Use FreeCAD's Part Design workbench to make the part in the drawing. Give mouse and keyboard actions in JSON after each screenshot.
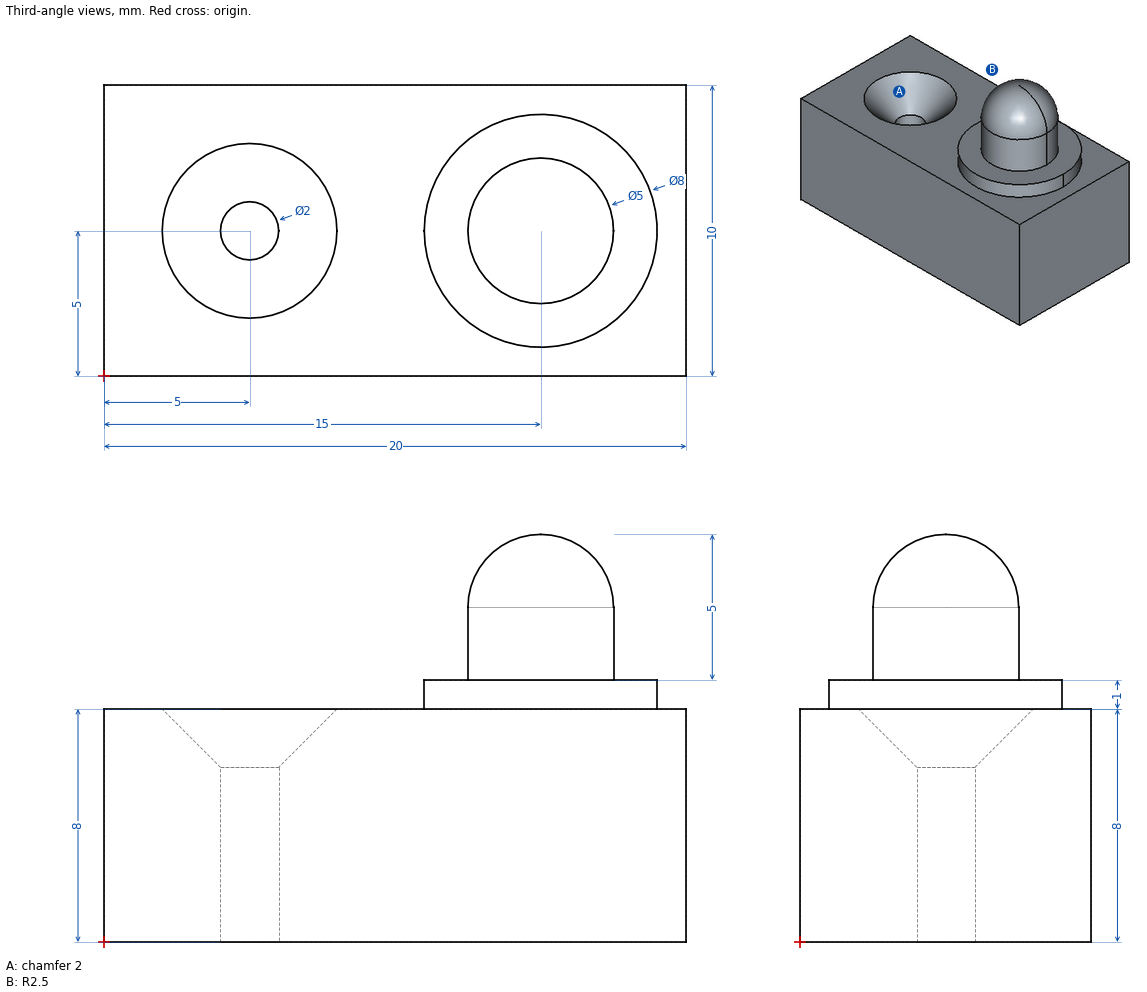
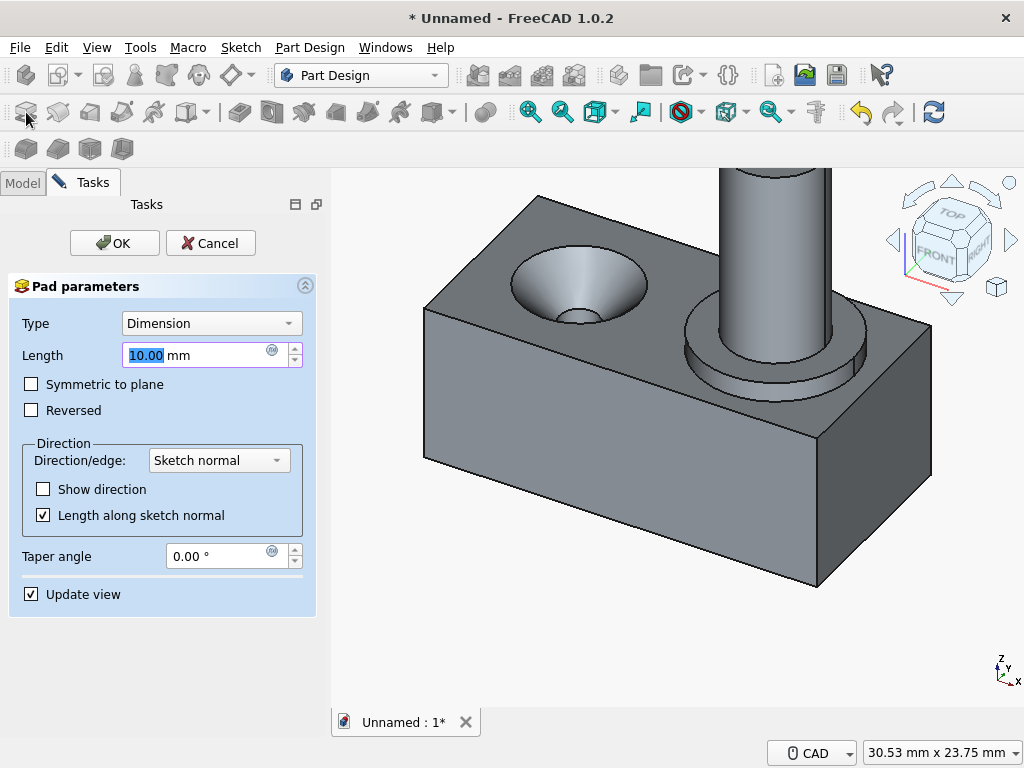
{"action": "type", "text": "5"}
{"action": "key", "text": "Tab"}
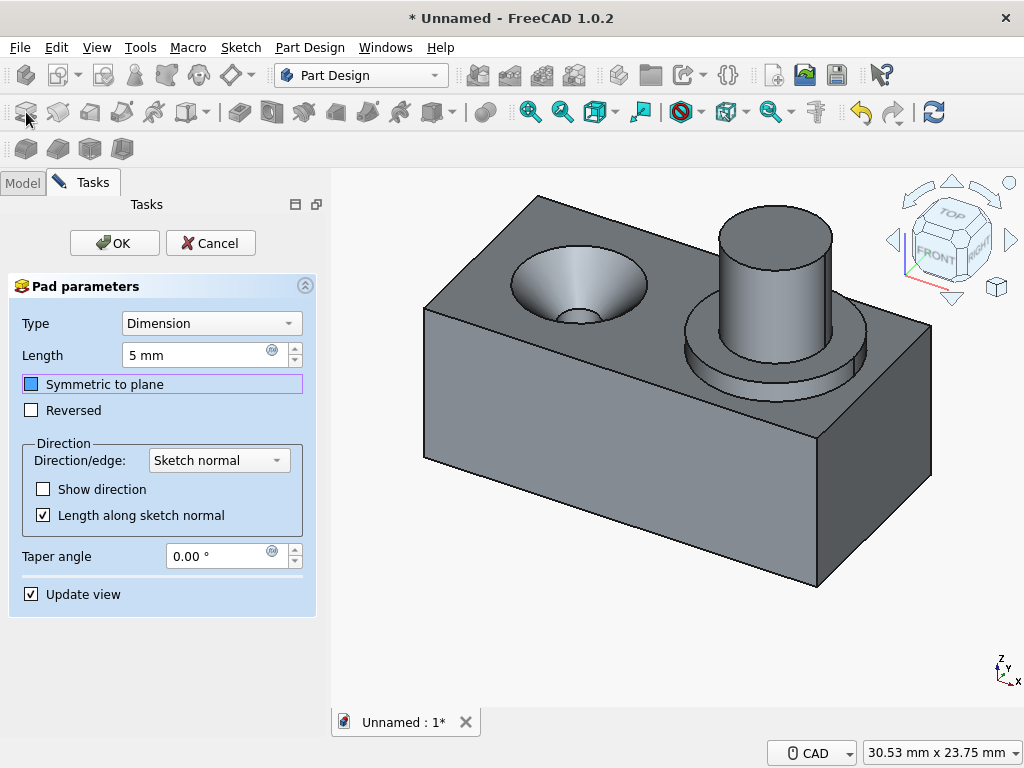
{"action": "left_click", "coordinate": [115, 243]}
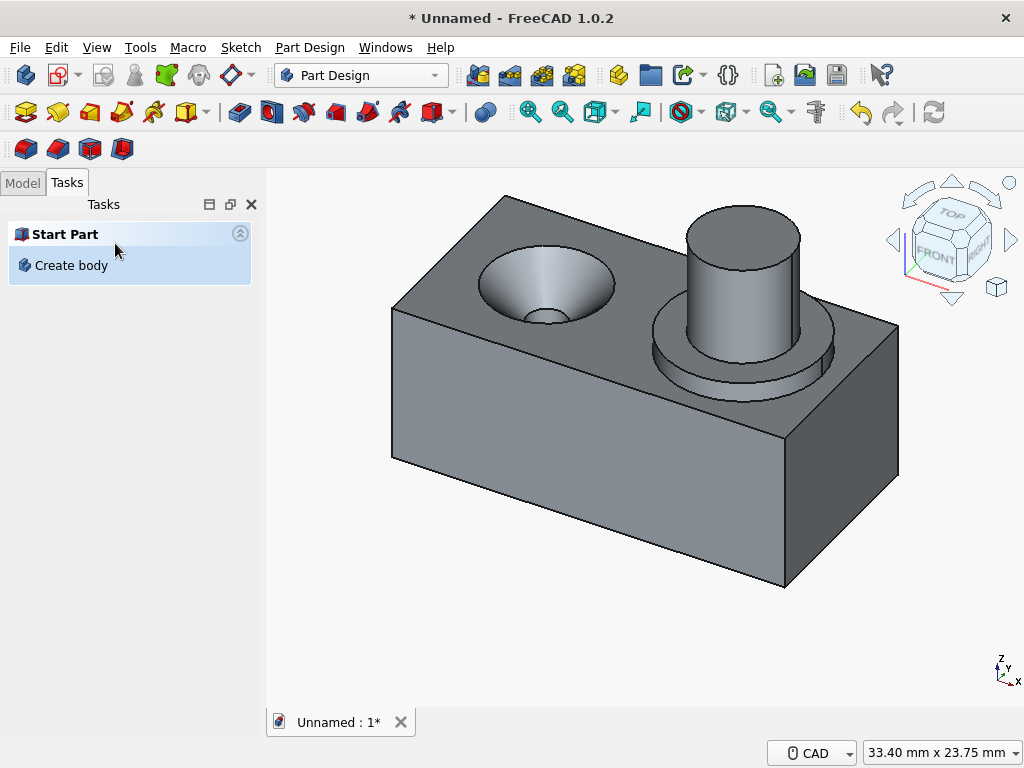
{"action": "left_click", "coordinate": [532, 112]}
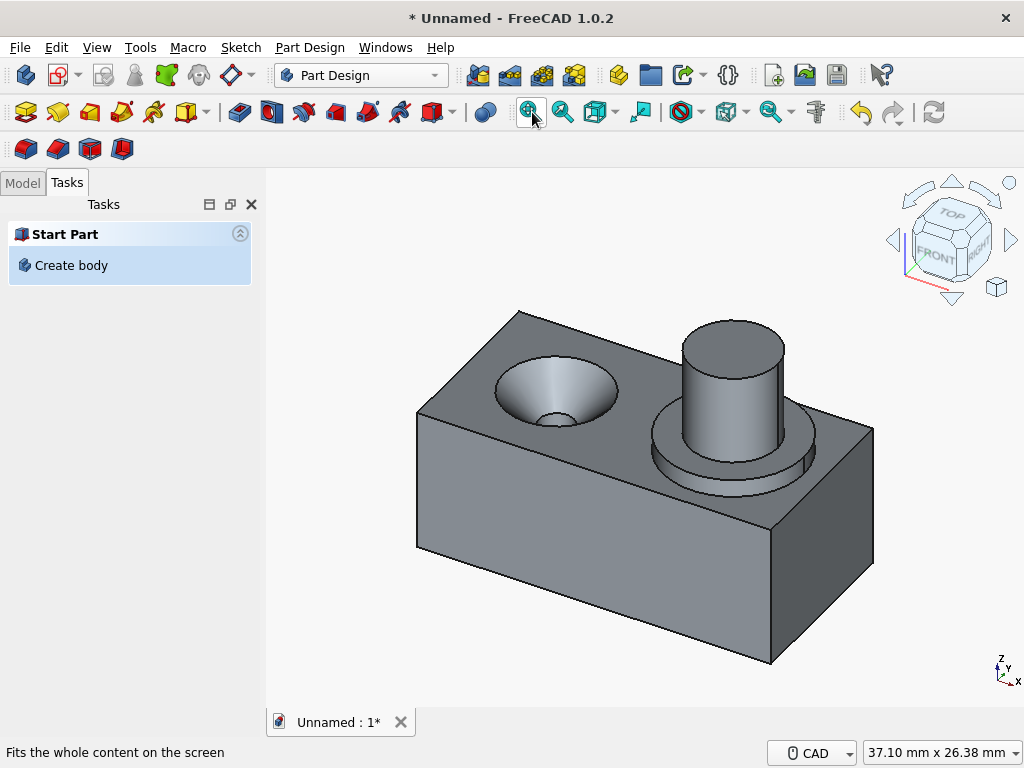
{"action": "left_click", "coordinate": [683, 352]}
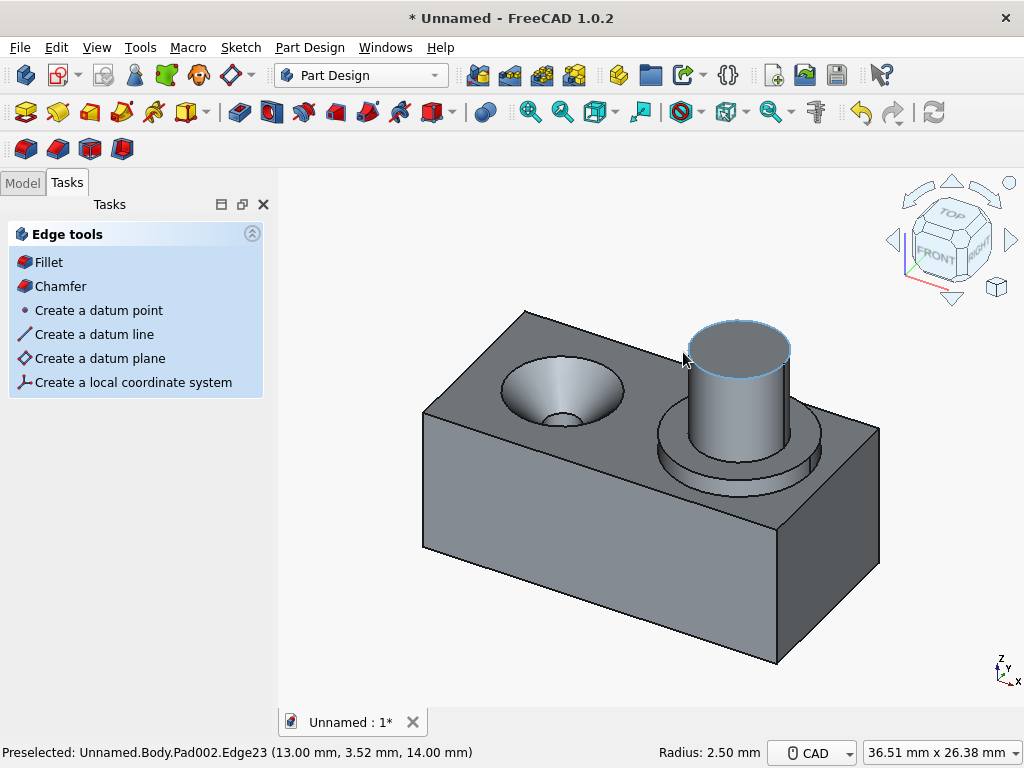
{"action": "left_click", "coordinate": [26, 150]}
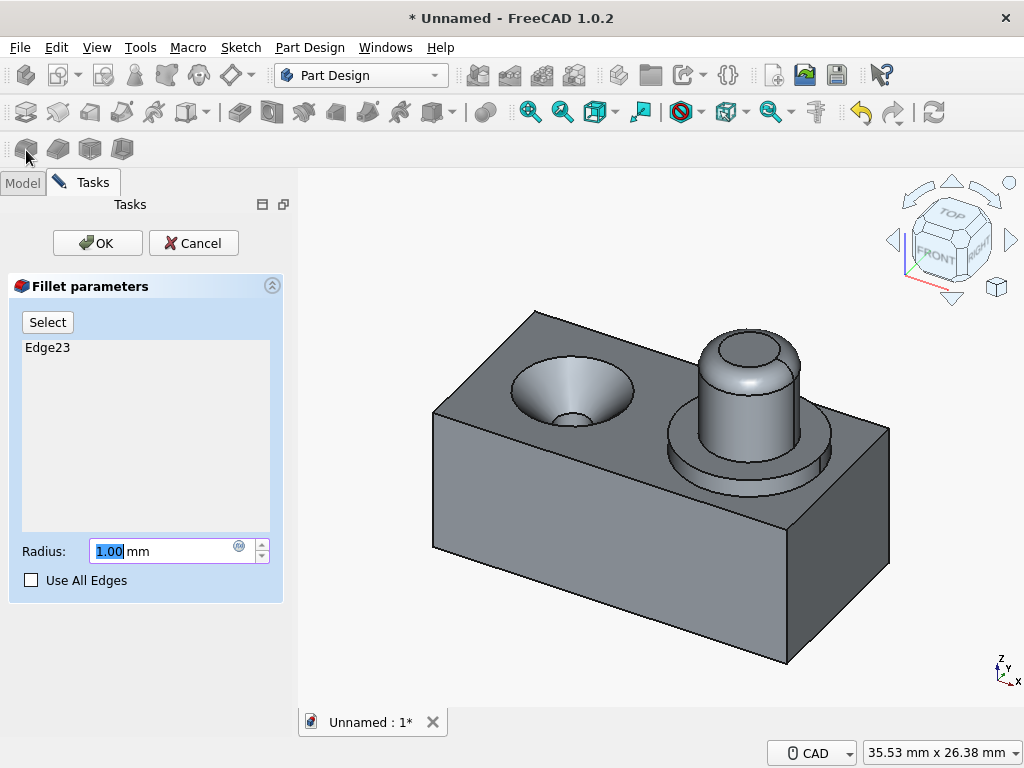
{"action": "type", "text": "2.5"}
{"action": "key", "text": "Tab"}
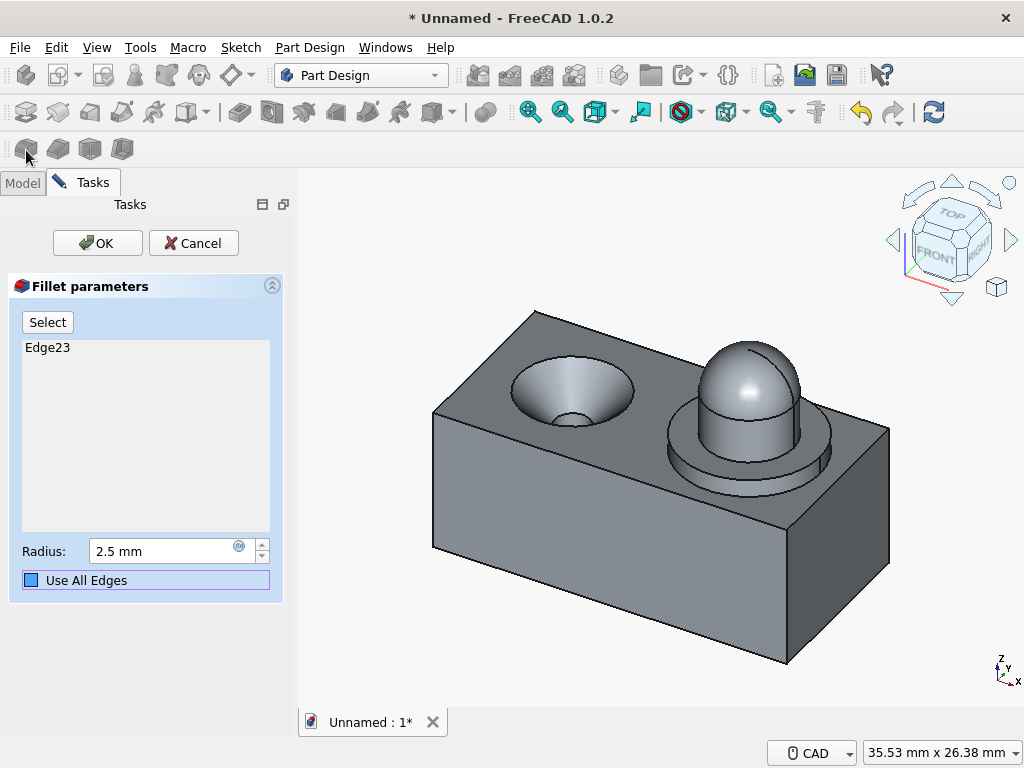
{"action": "left_click", "coordinate": [98, 243]}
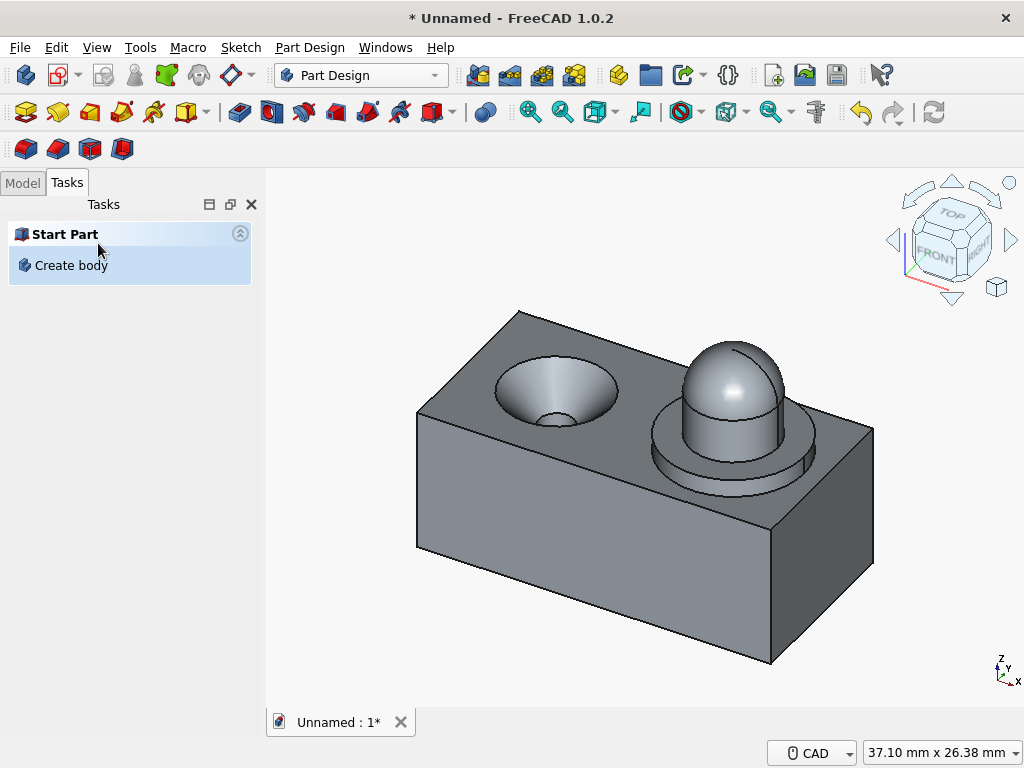
{"action": "key", "text": "0"}